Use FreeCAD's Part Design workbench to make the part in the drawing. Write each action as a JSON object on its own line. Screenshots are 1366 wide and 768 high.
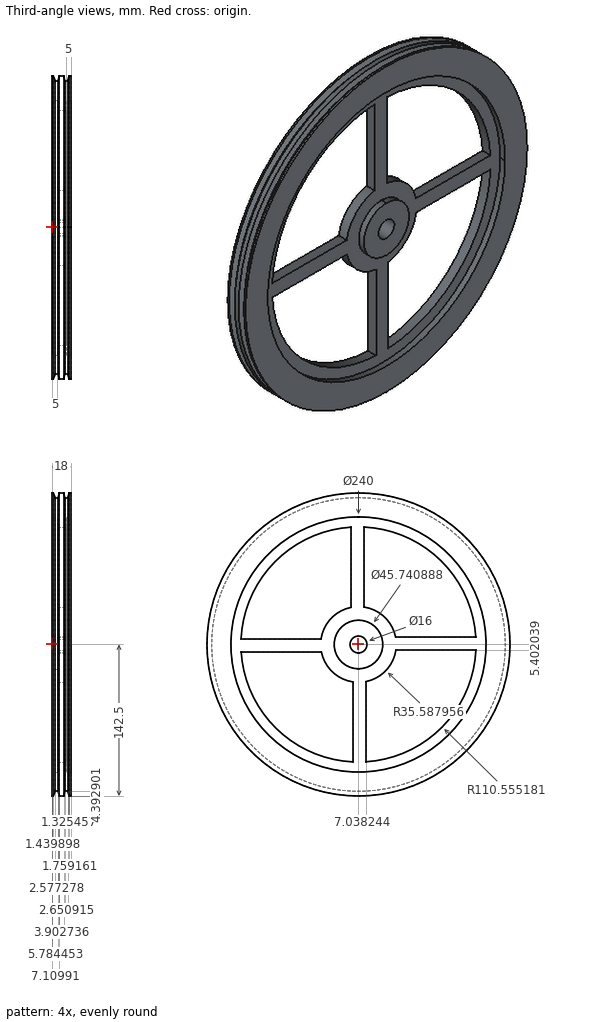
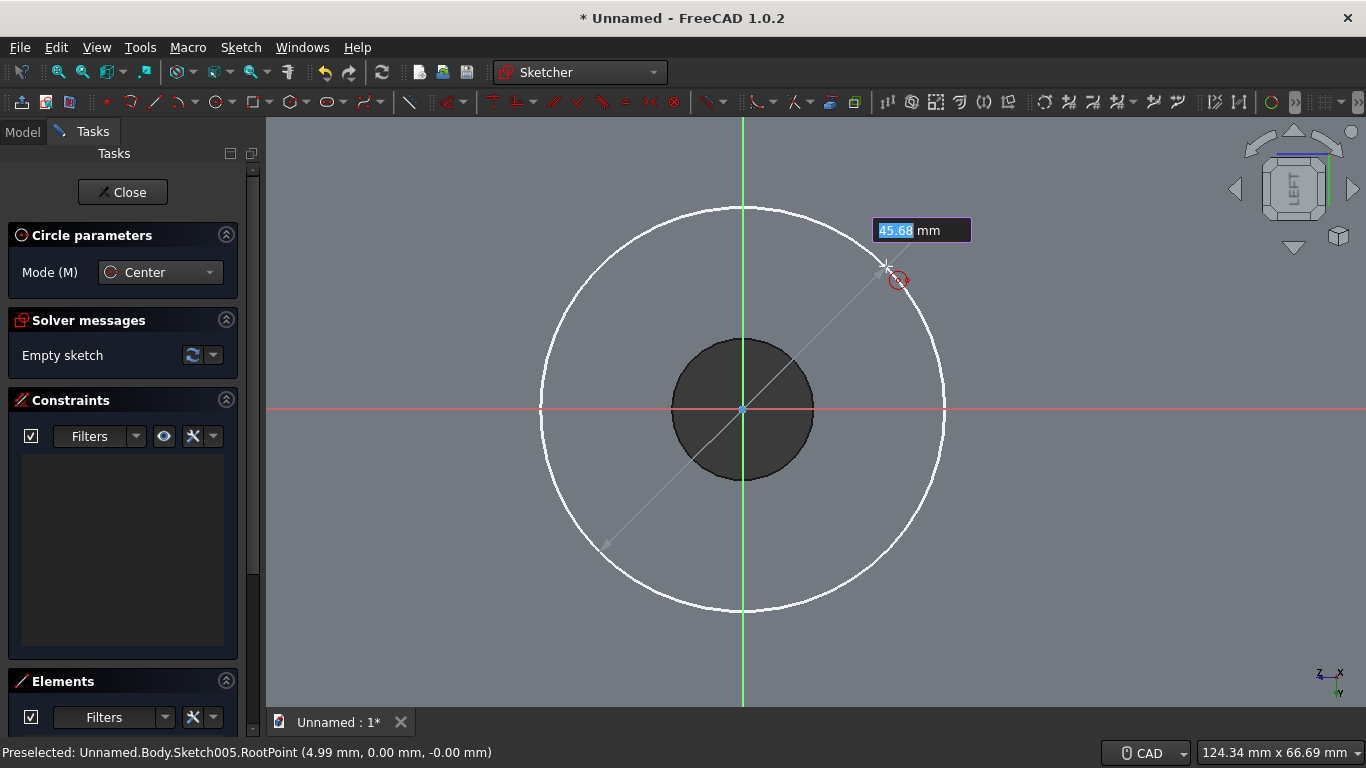
{"action": "type", "text": "45.740888"}
{"action": "key", "text": "Return"}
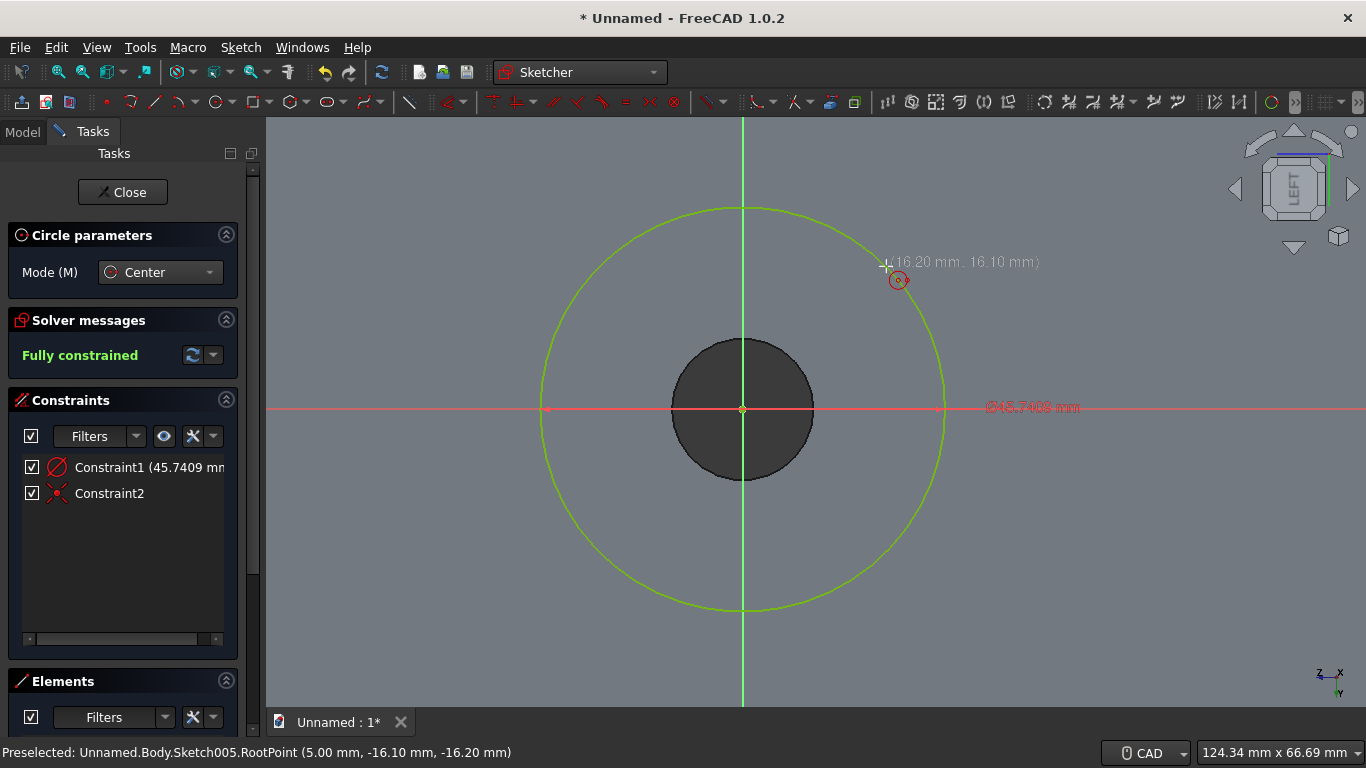
{"action": "left_click", "coordinate": [743, 409]}
{"action": "mouse_move", "coordinate": [793, 359]}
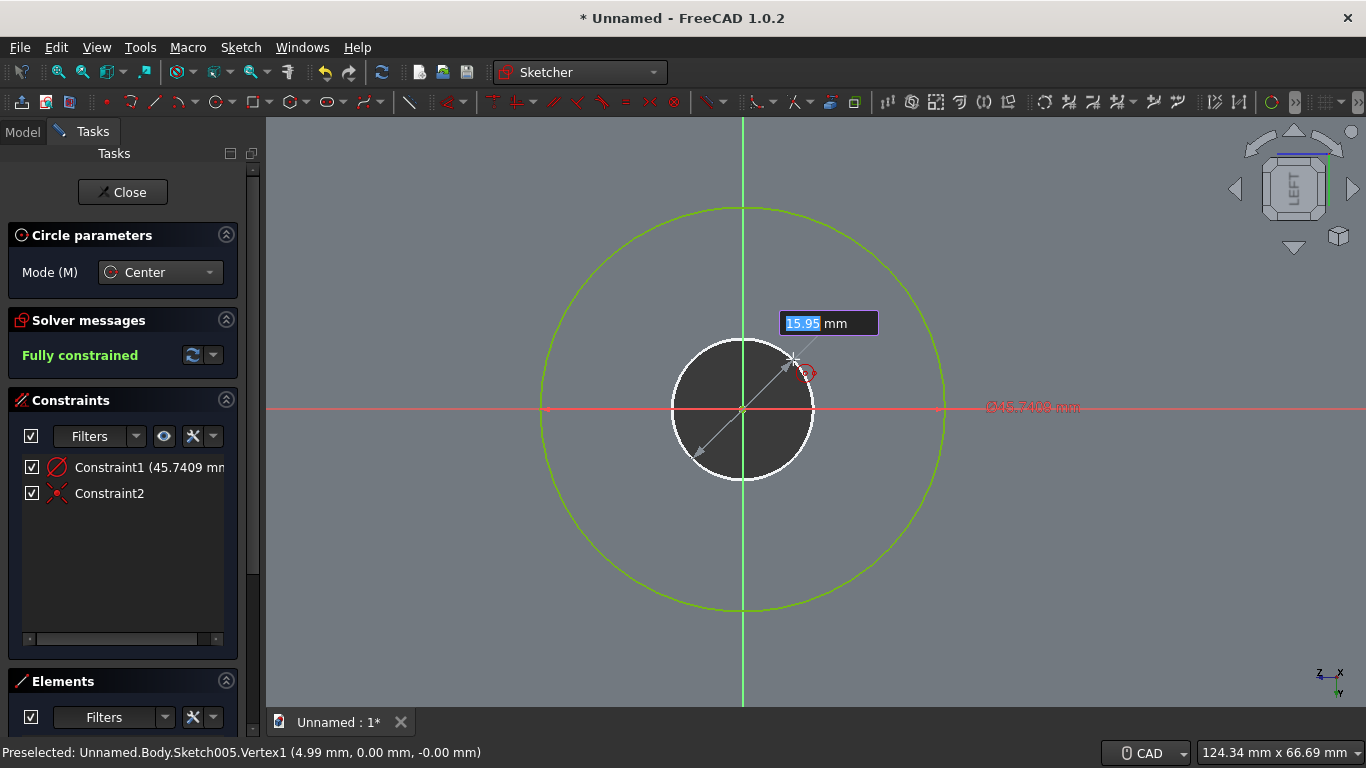
{"action": "type", "text": "16"}
{"action": "key", "text": "Return"}
{"action": "key", "text": "Escape"}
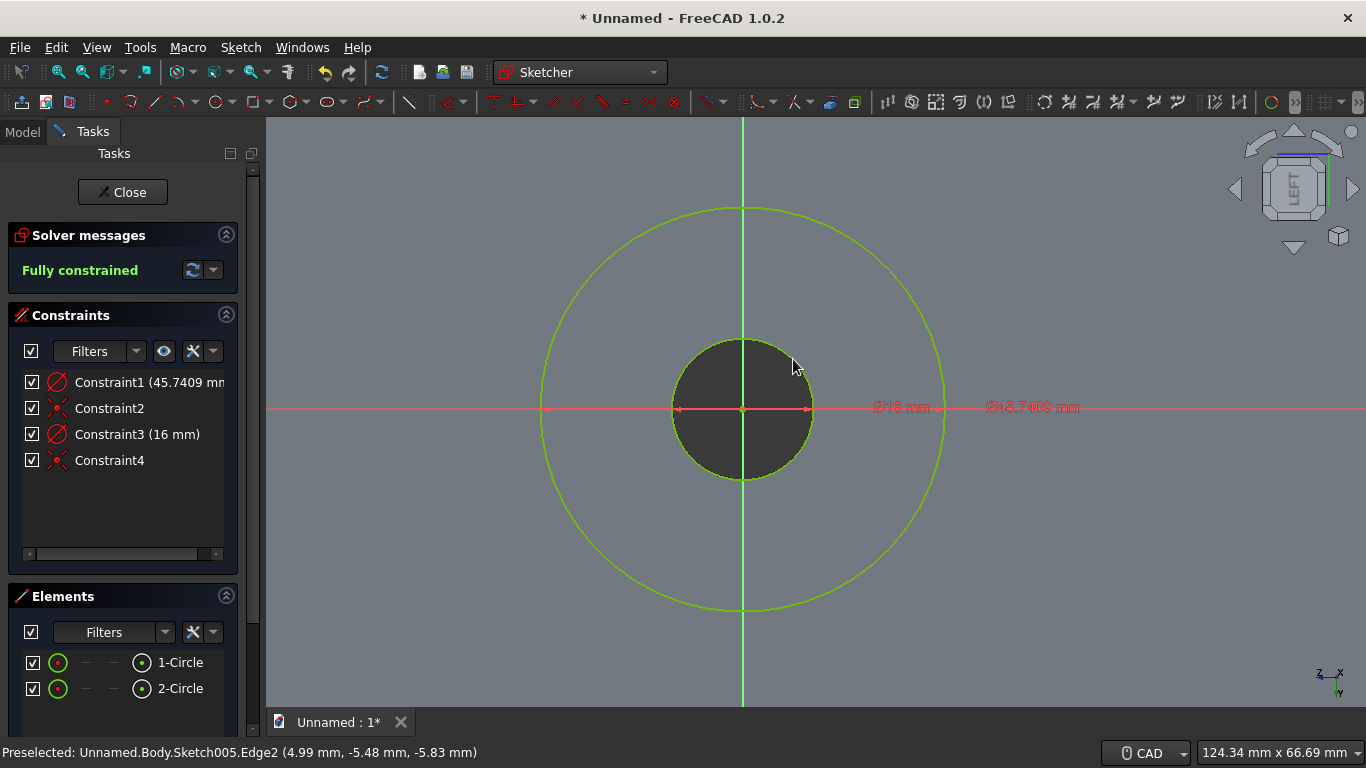
{"action": "left_click", "coordinate": [123, 192]}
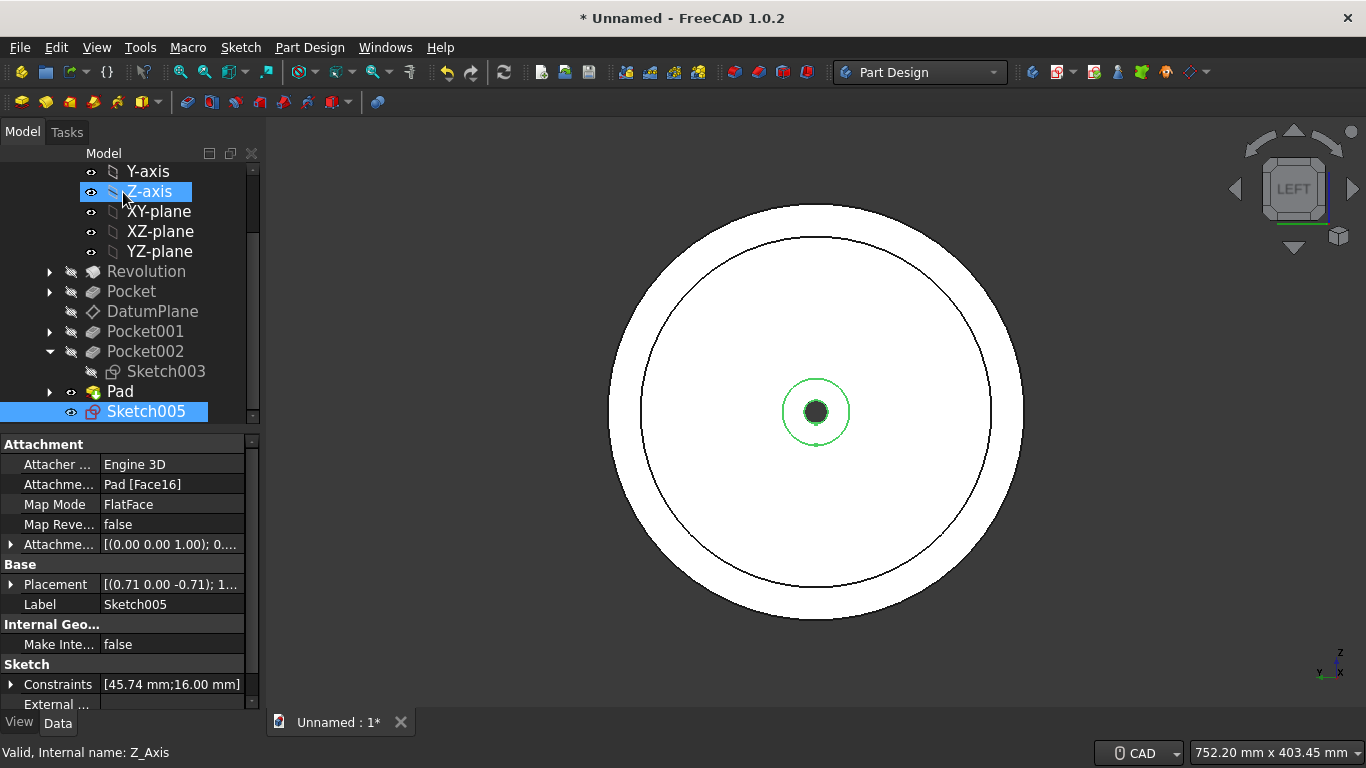
{"action": "left_click", "coordinate": [22, 102]}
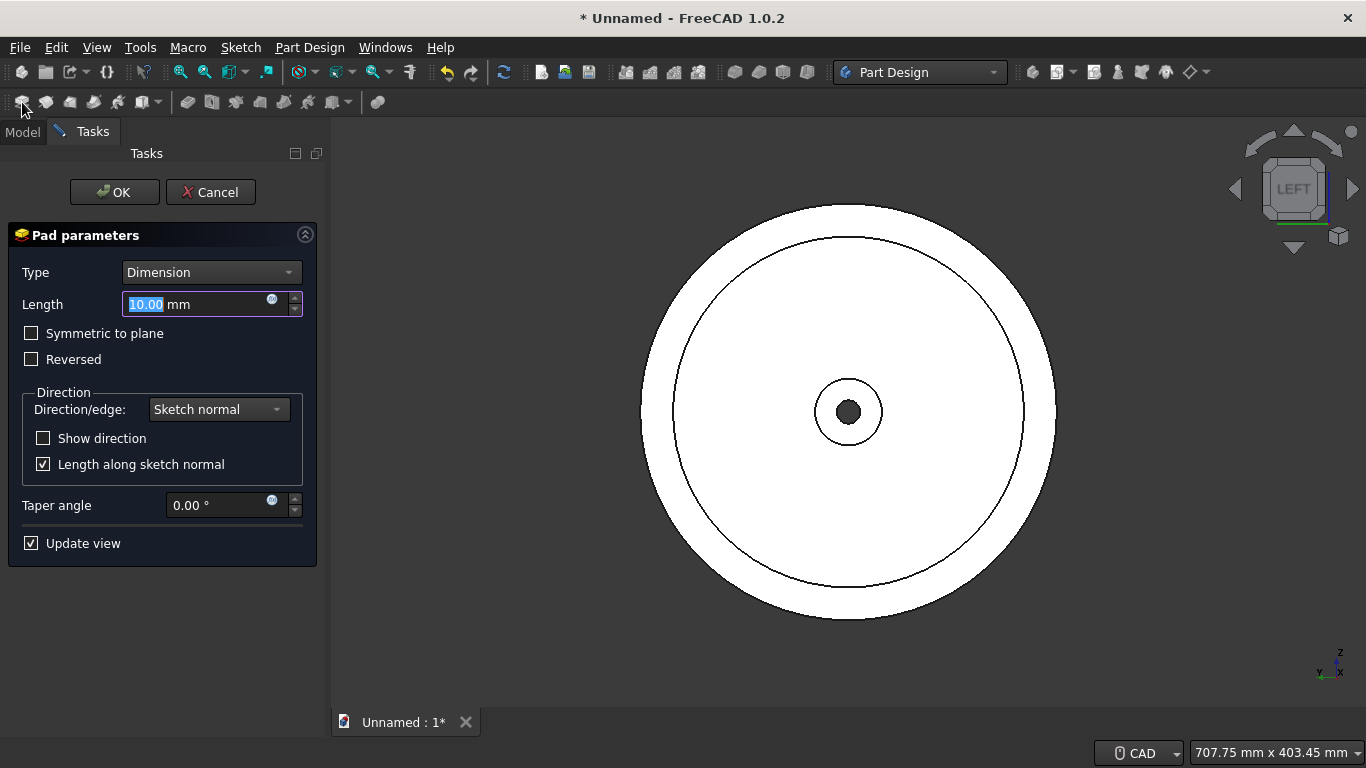
{"action": "type", "text": "5"}
{"action": "key", "text": "Tab"}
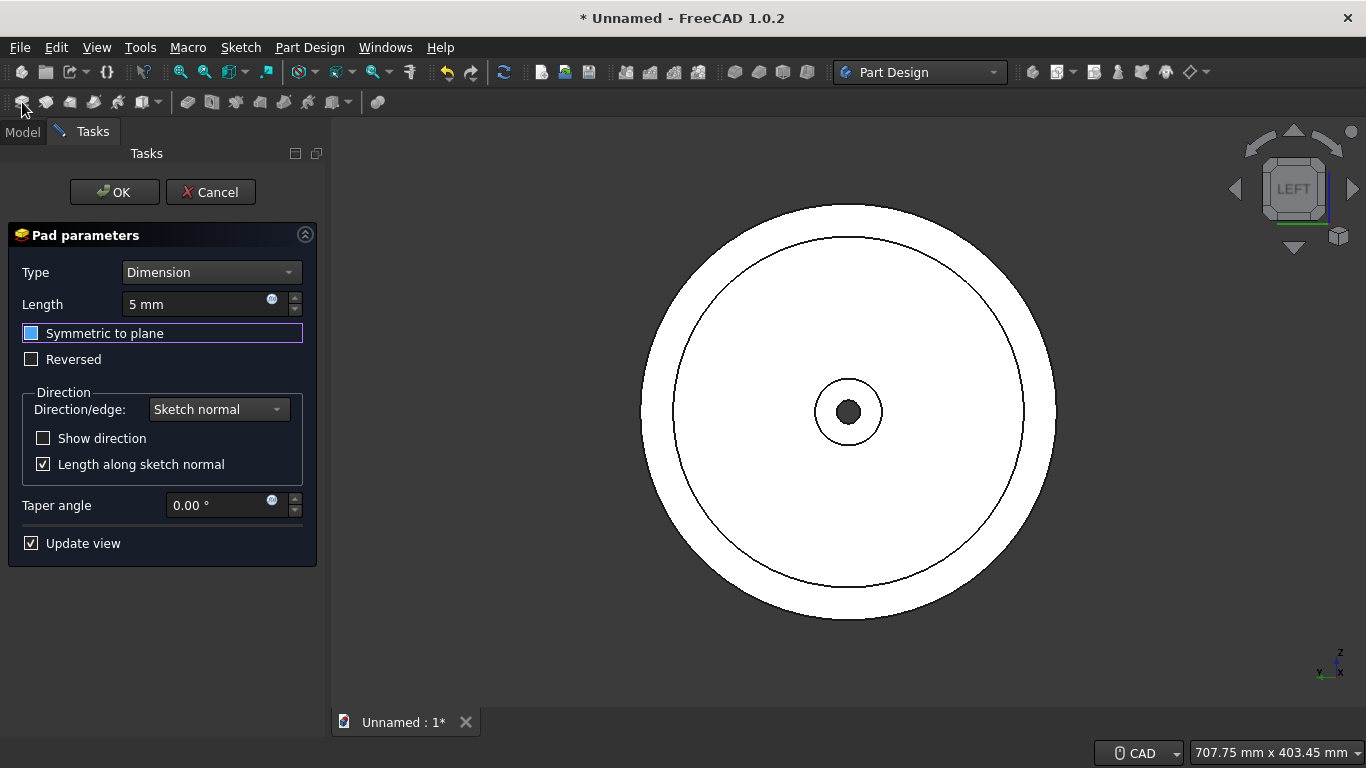
{"action": "left_click", "coordinate": [115, 192]}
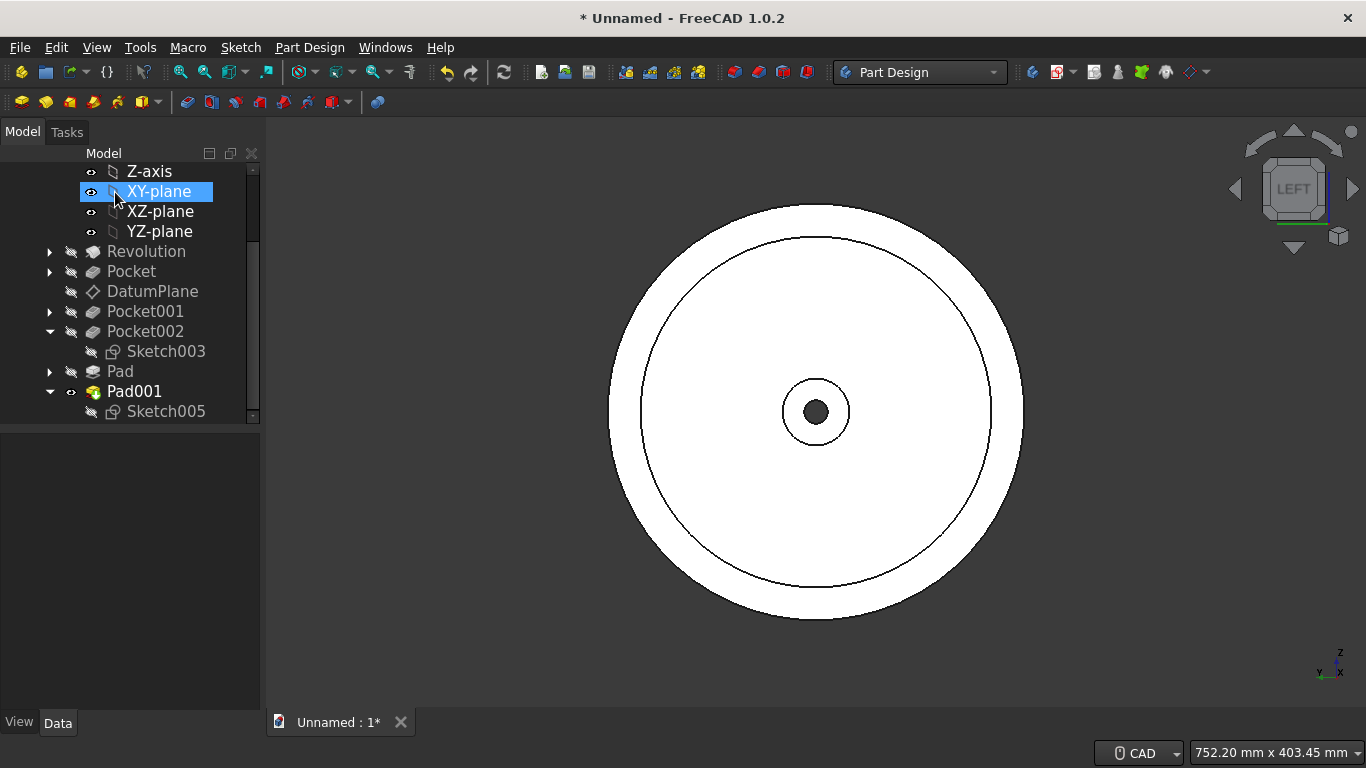
{"action": "left_click", "coordinate": [816, 311]}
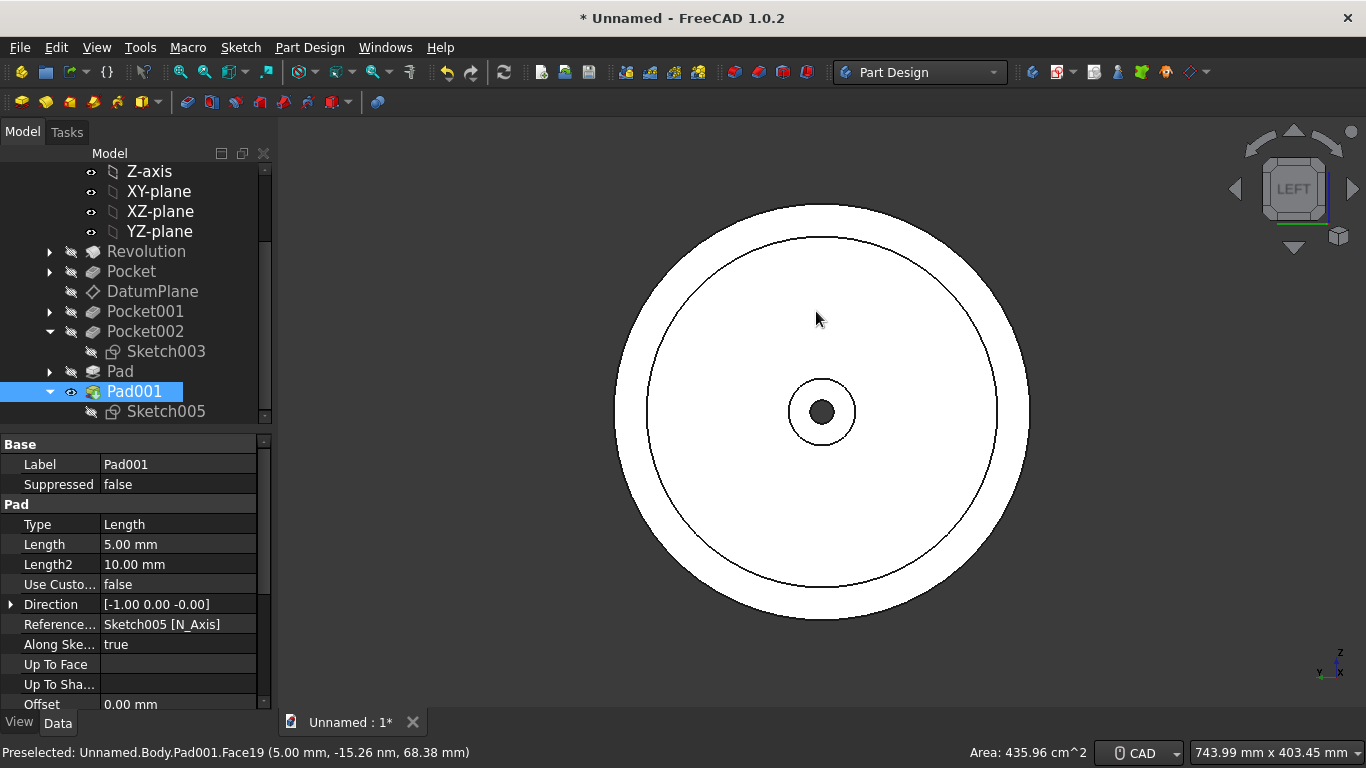
{"action": "left_click", "coordinate": [1058, 72]}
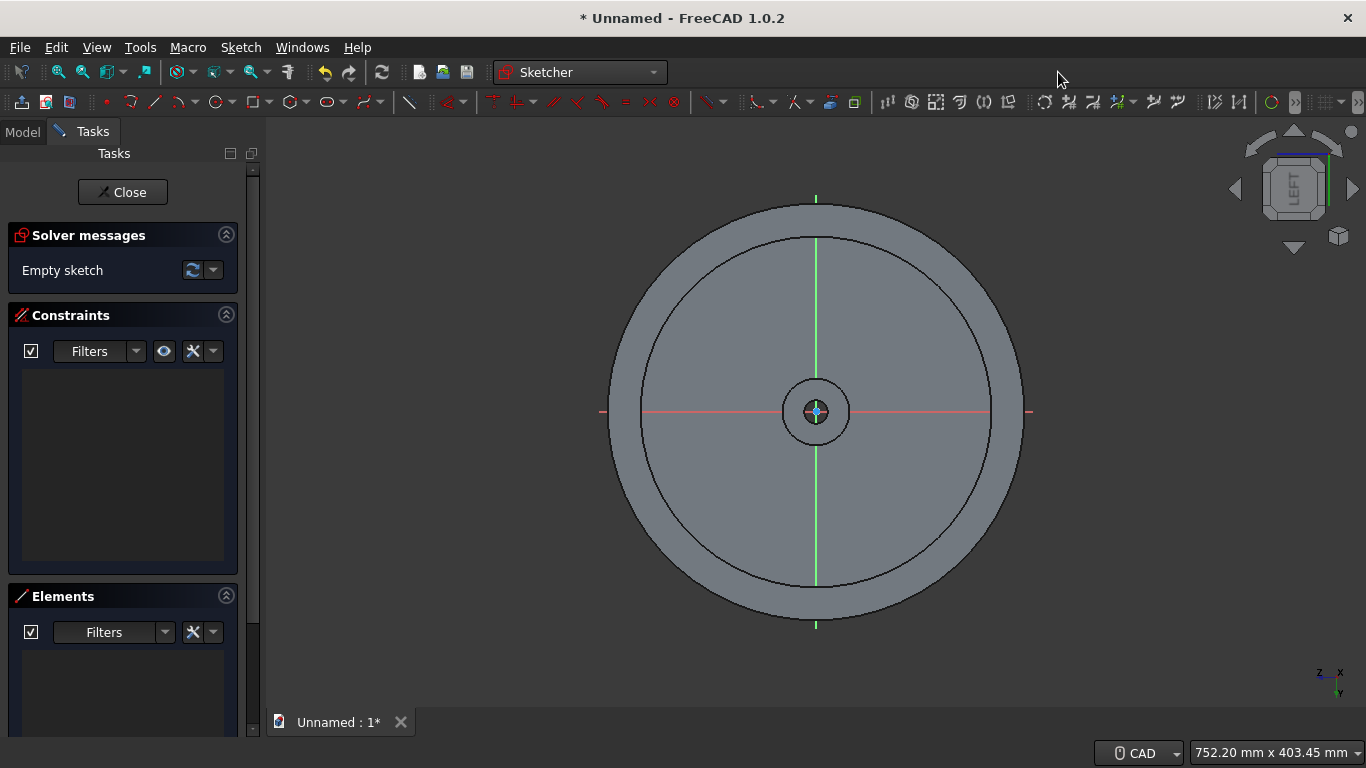
{"action": "left_click", "coordinate": [70, 102]}